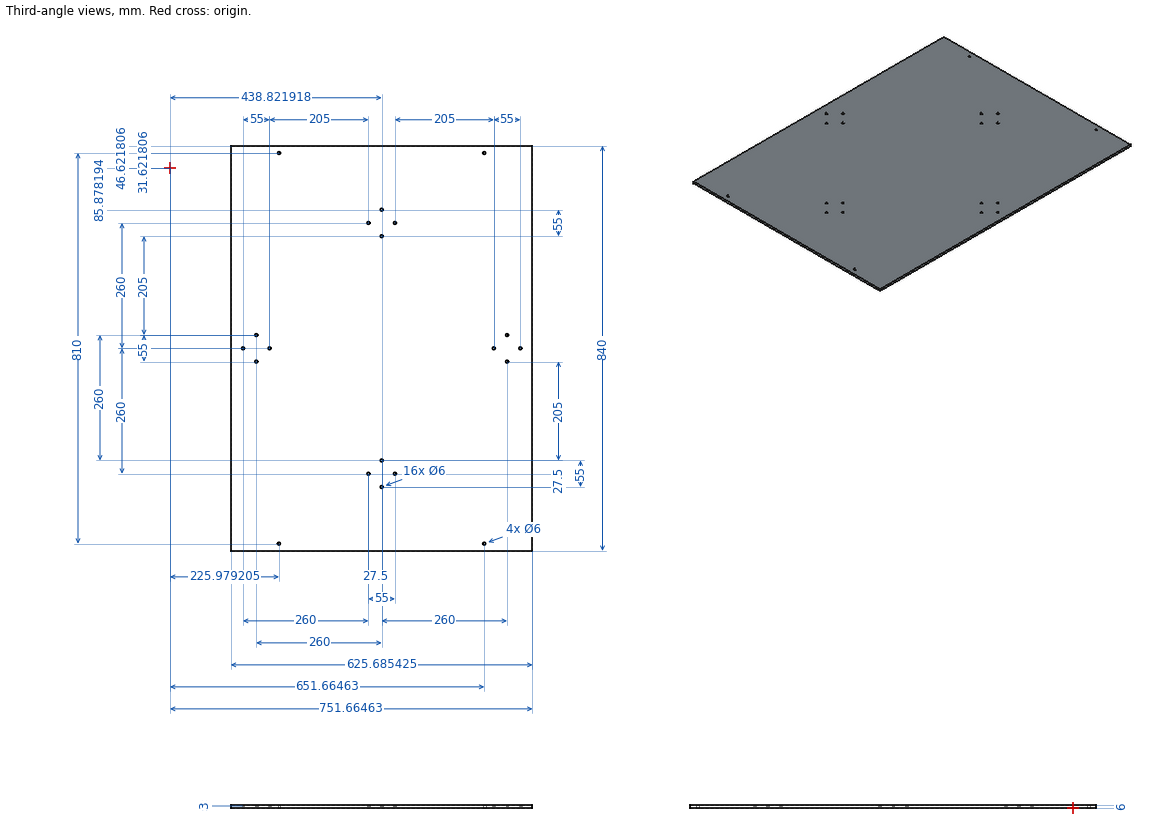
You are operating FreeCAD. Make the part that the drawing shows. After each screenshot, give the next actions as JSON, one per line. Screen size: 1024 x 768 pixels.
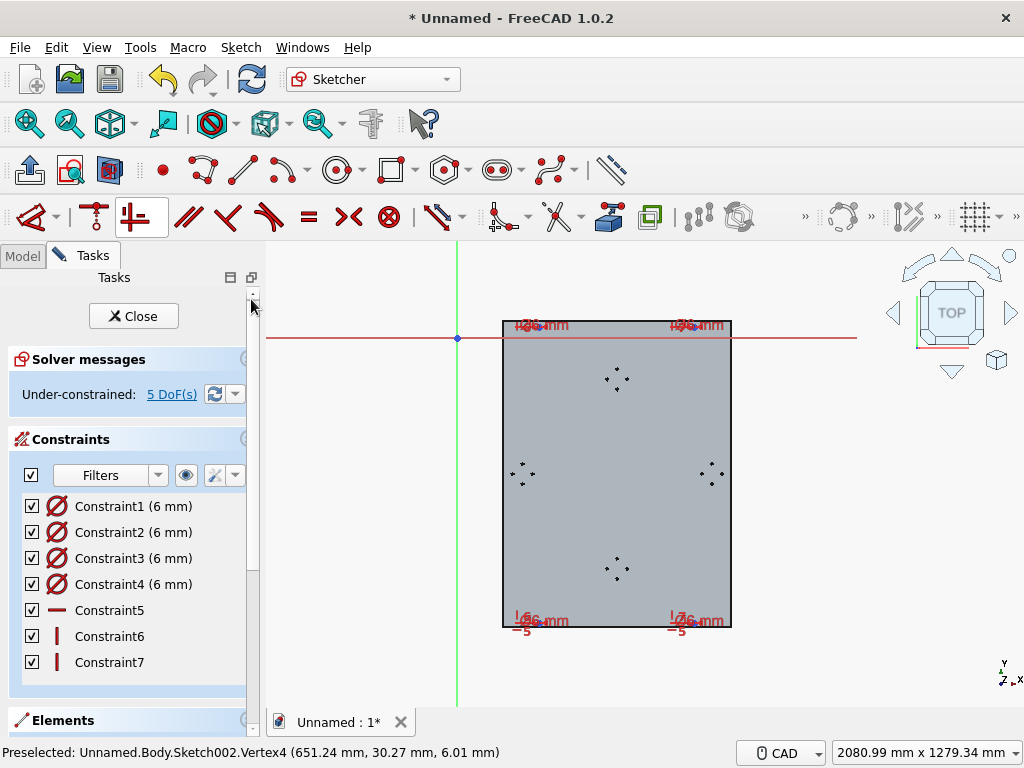
{"action": "left_click", "coordinate": [540, 327]}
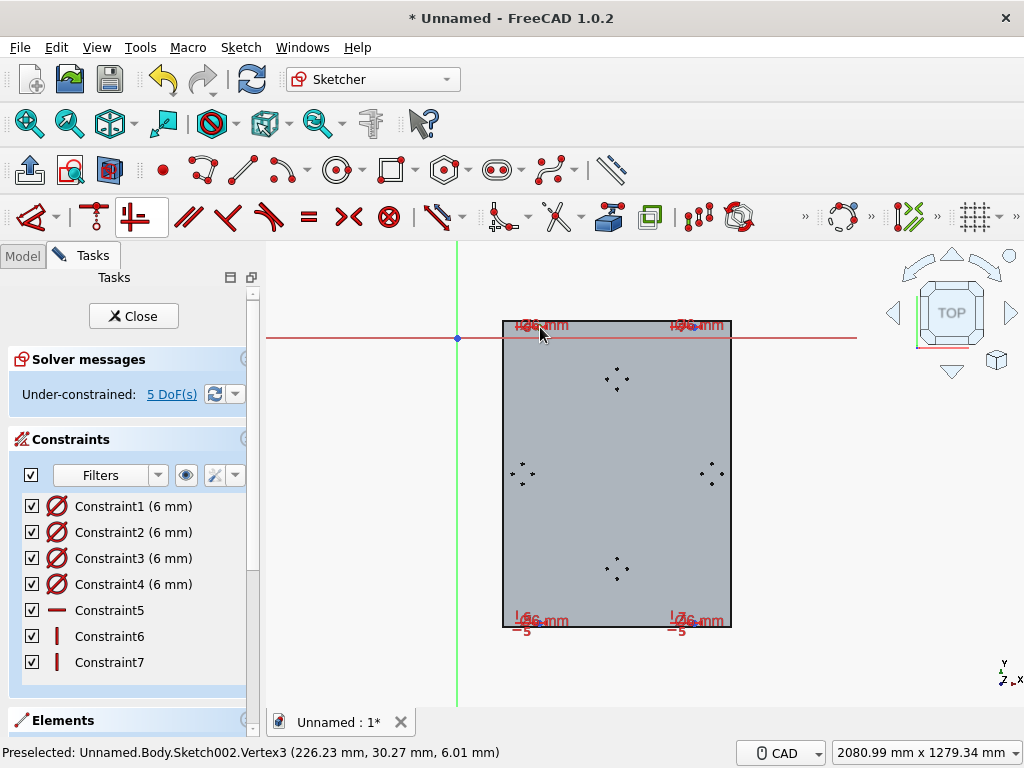
{"action": "left_click", "coordinate": [695, 327]}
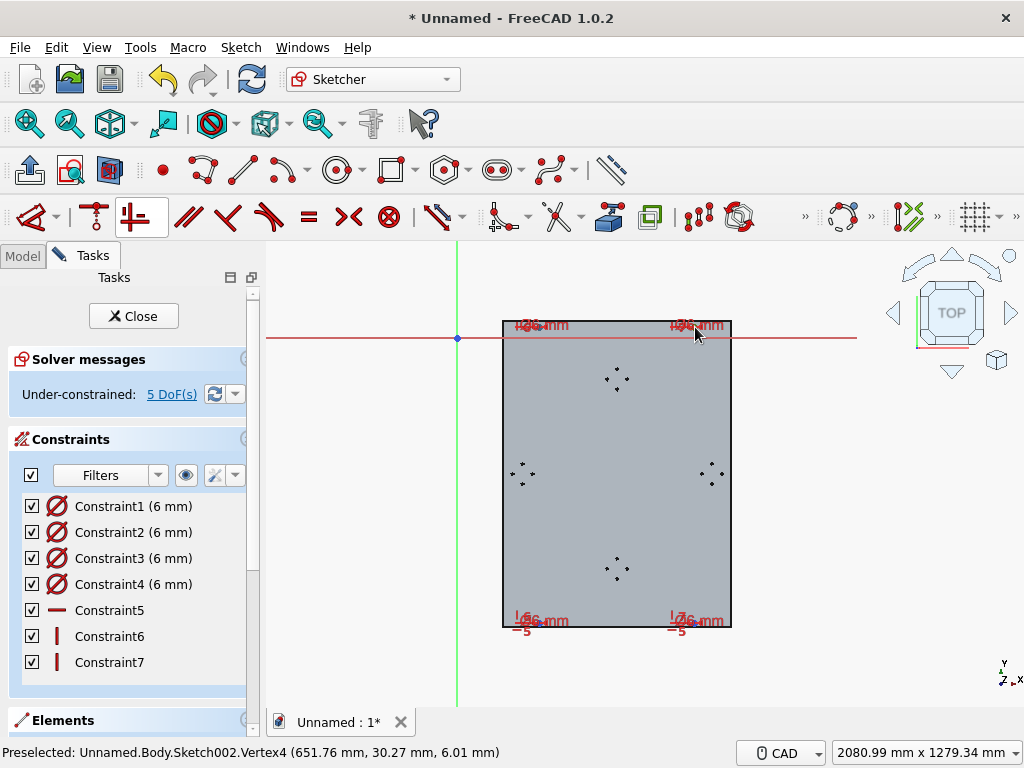
{"action": "key", "text": "h"}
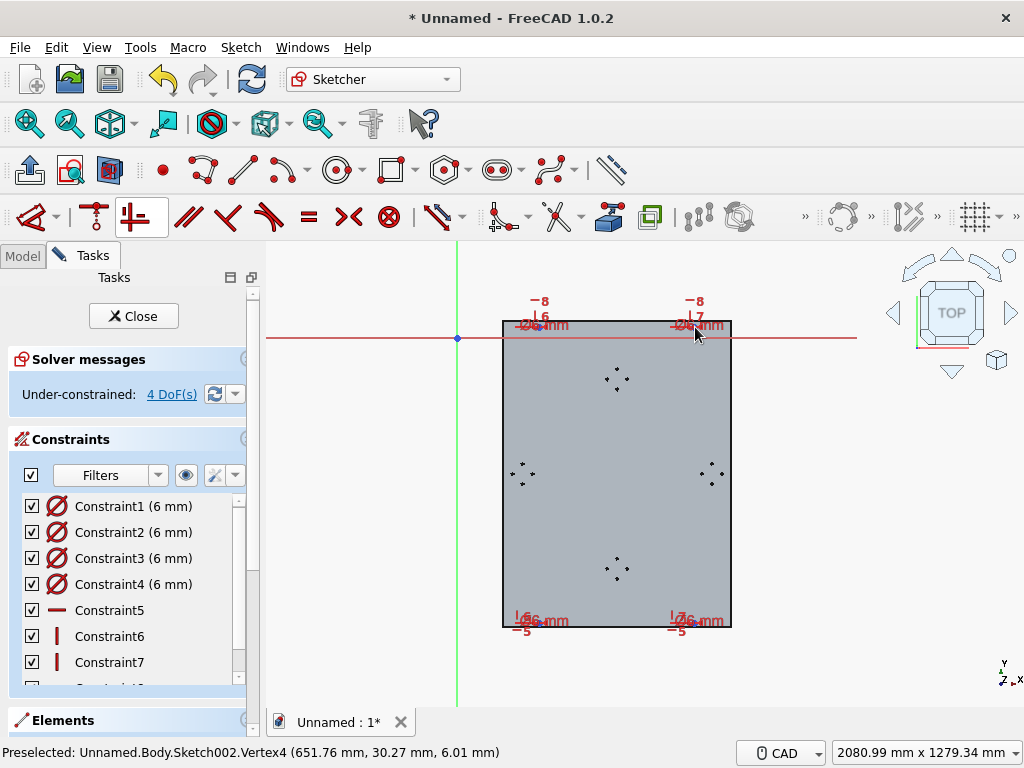
{"action": "left_click", "coordinate": [32, 218]}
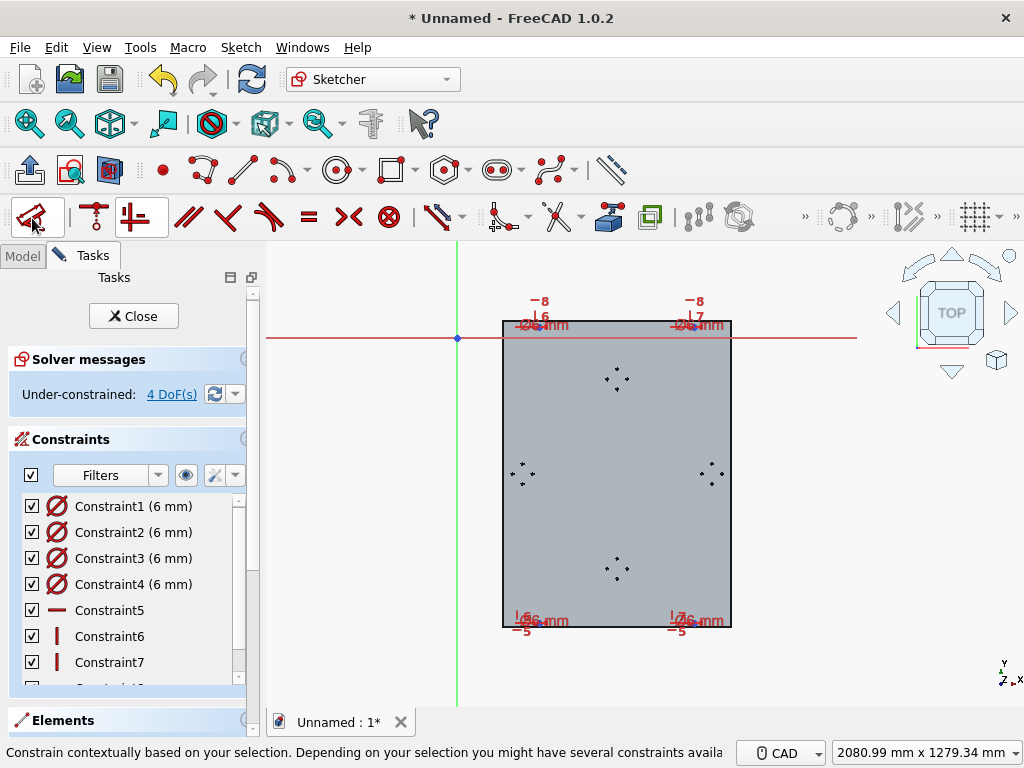
{"action": "left_click", "coordinate": [540, 623]}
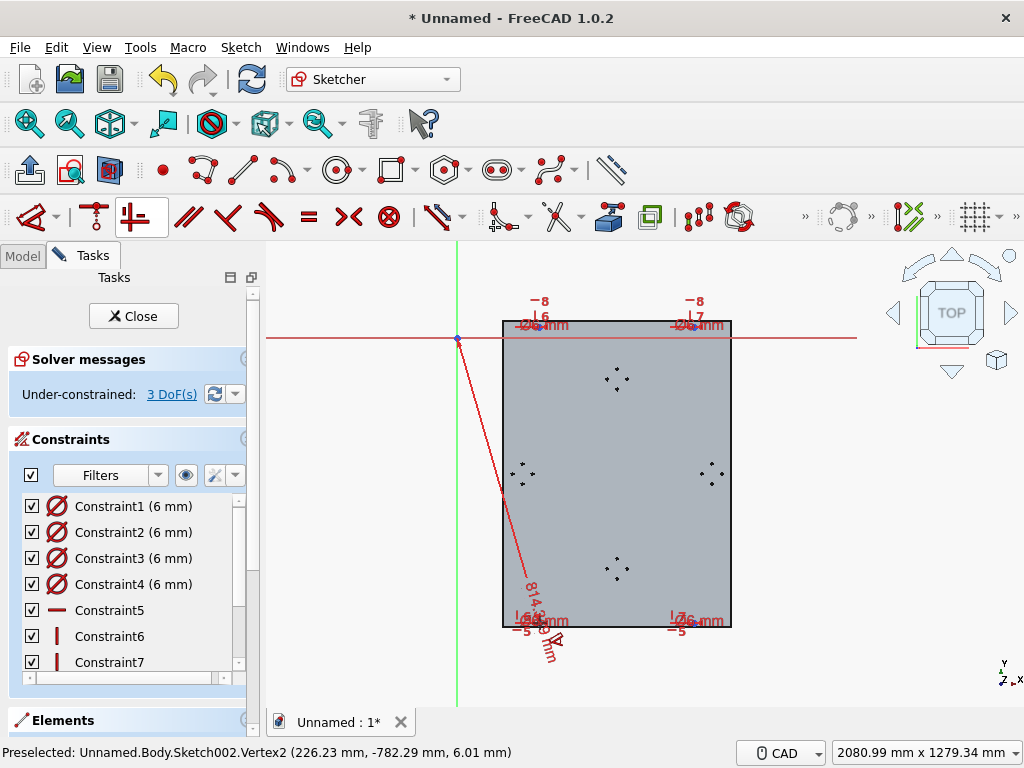
{"action": "left_click", "coordinate": [540, 327]}
{"action": "left_click", "coordinate": [506, 475]}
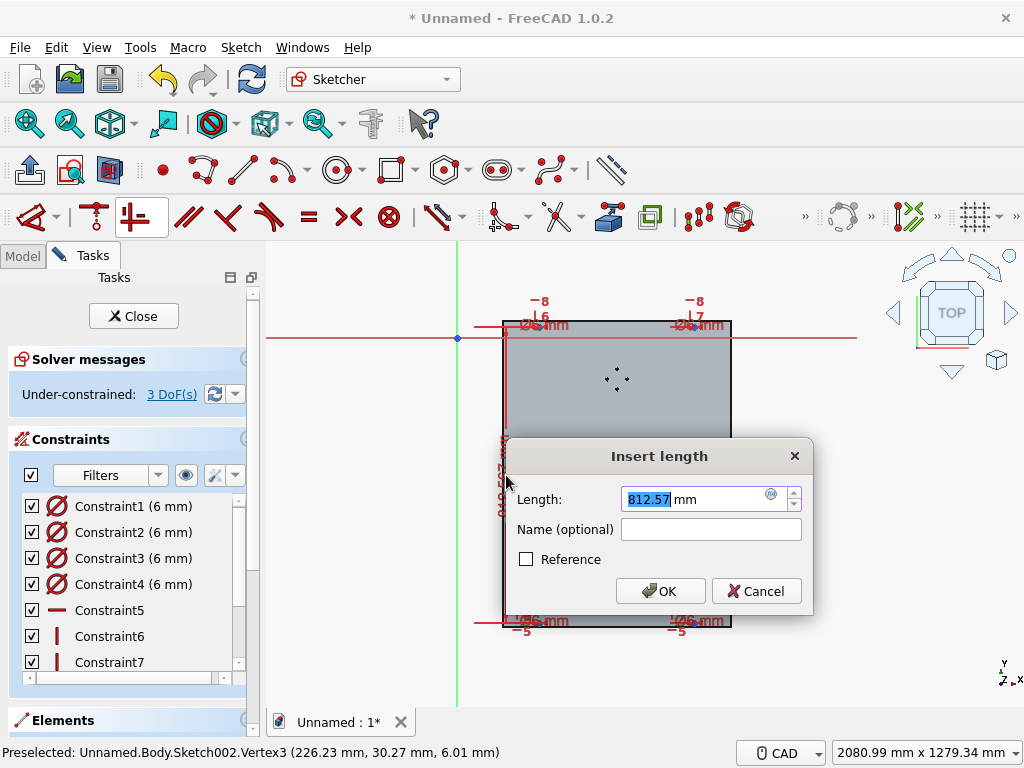
{"action": "type", "text": "810"}
{"action": "key", "text": "Return"}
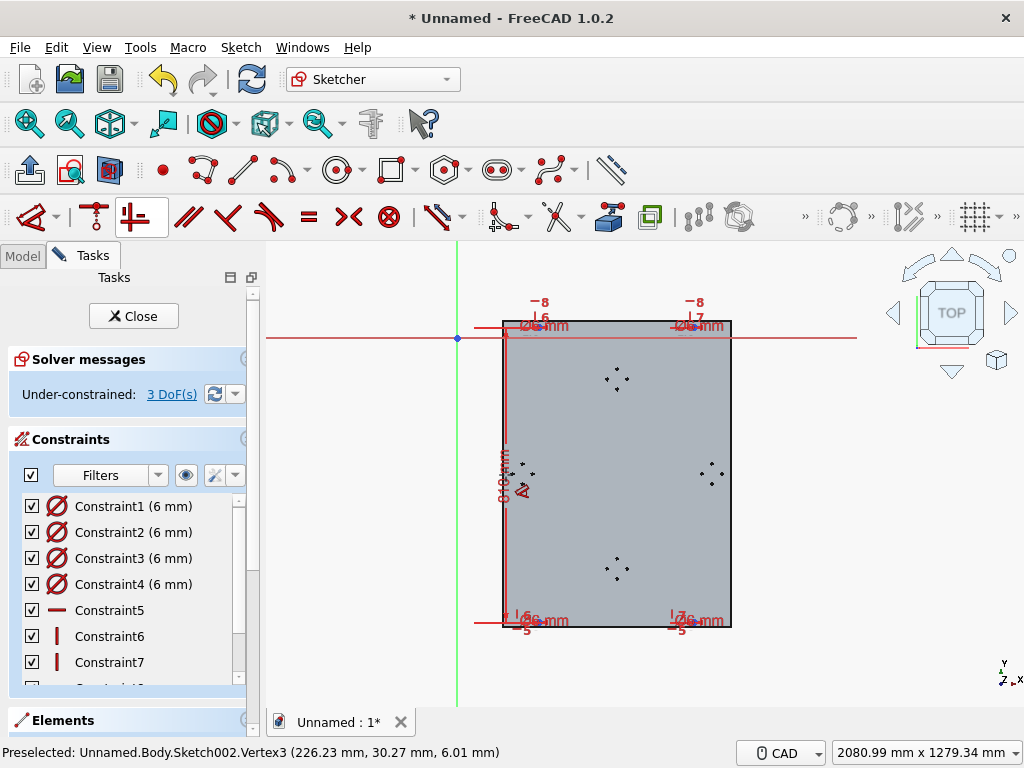
{"action": "left_click", "coordinate": [695, 623]}
{"action": "left_click", "coordinate": [576, 657]}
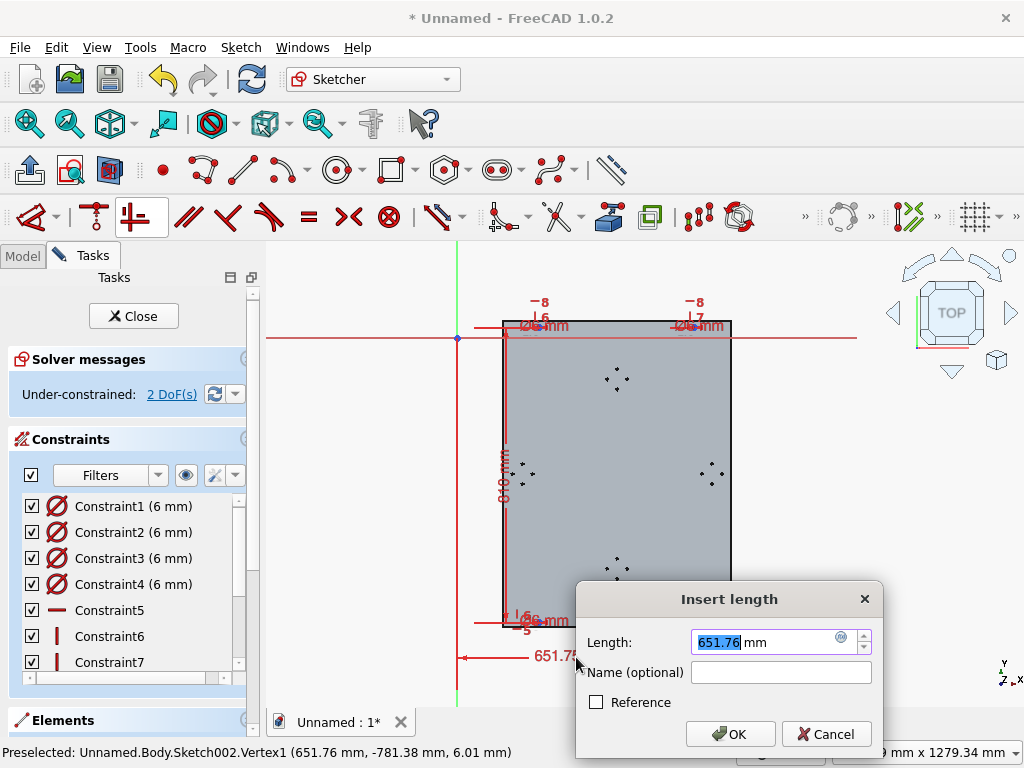
{"action": "type", "text": "651.66463"}
{"action": "key", "text": "Return"}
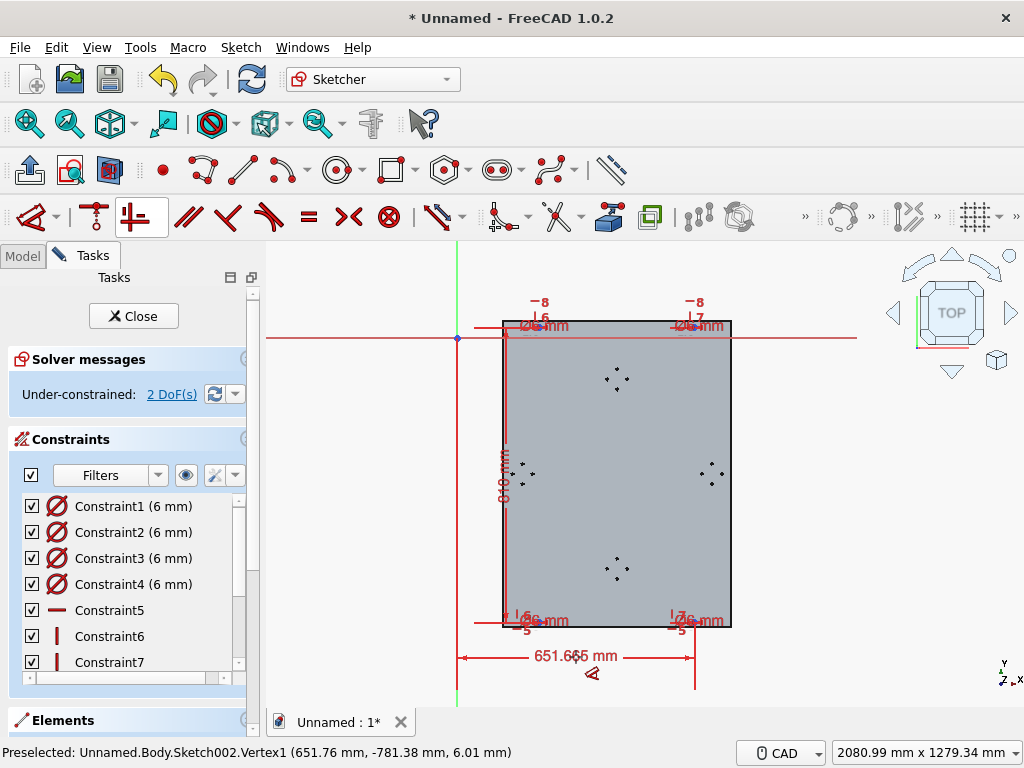
{"action": "scroll", "coordinate": [540, 328], "scroll_direction": "up", "scroll_amount": 7}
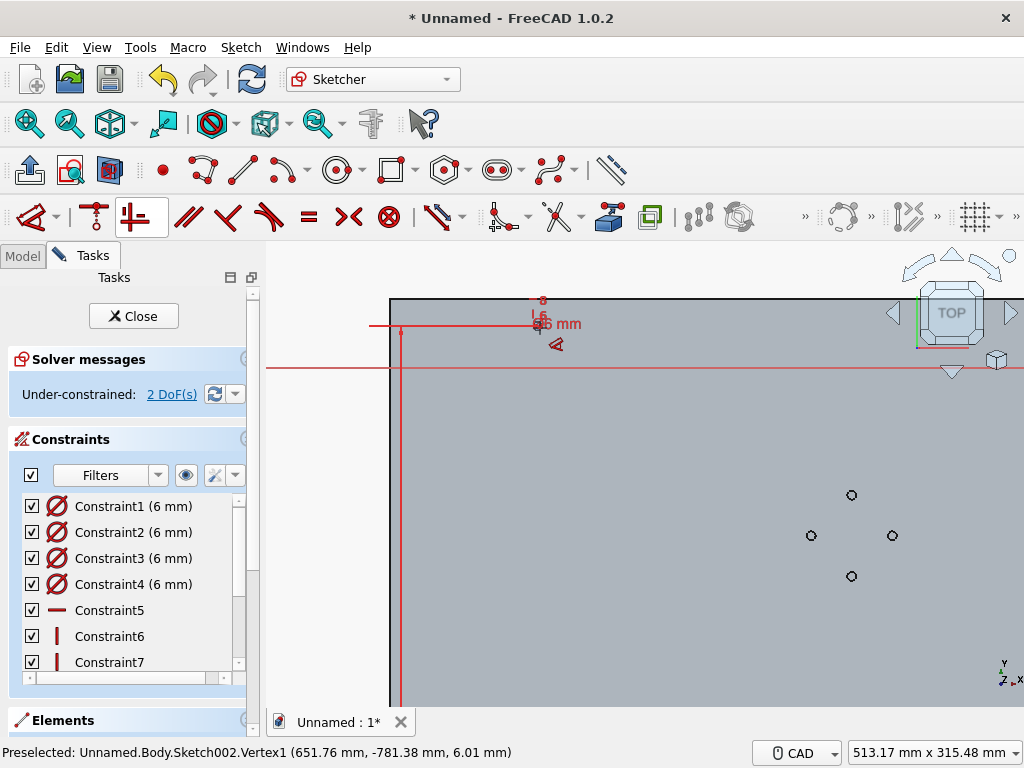
{"action": "left_click", "coordinate": [538, 326]}
{"action": "left_click", "coordinate": [572, 347]}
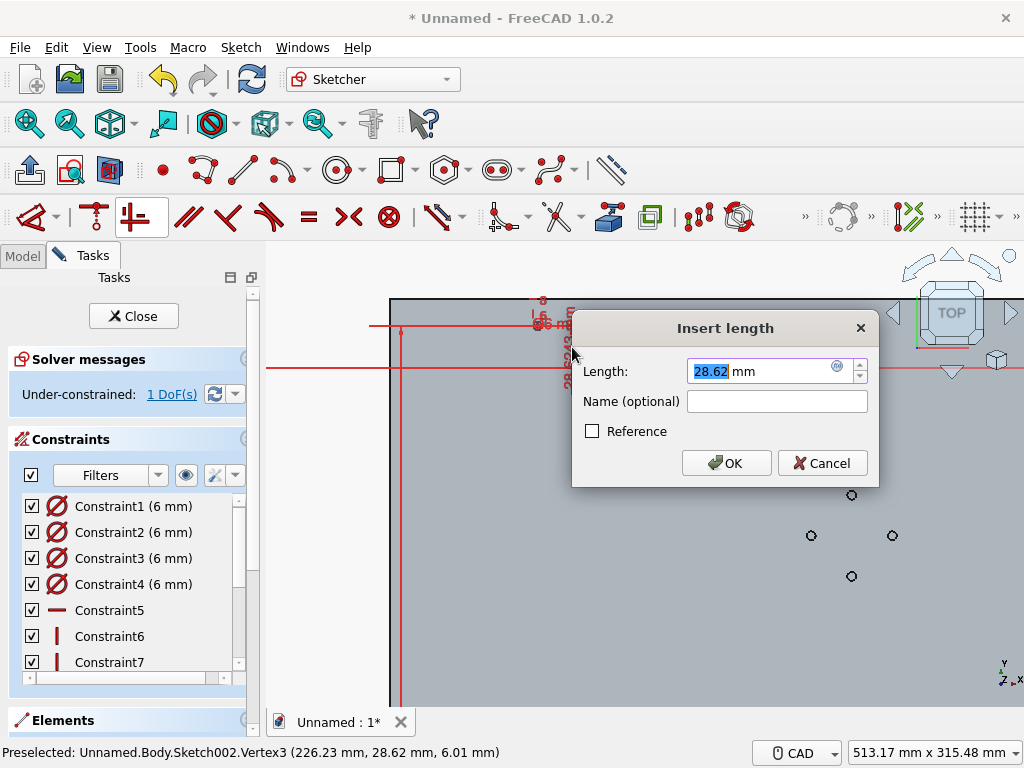
{"action": "type", "text": "31.621806"}
{"action": "key", "text": "Return"}